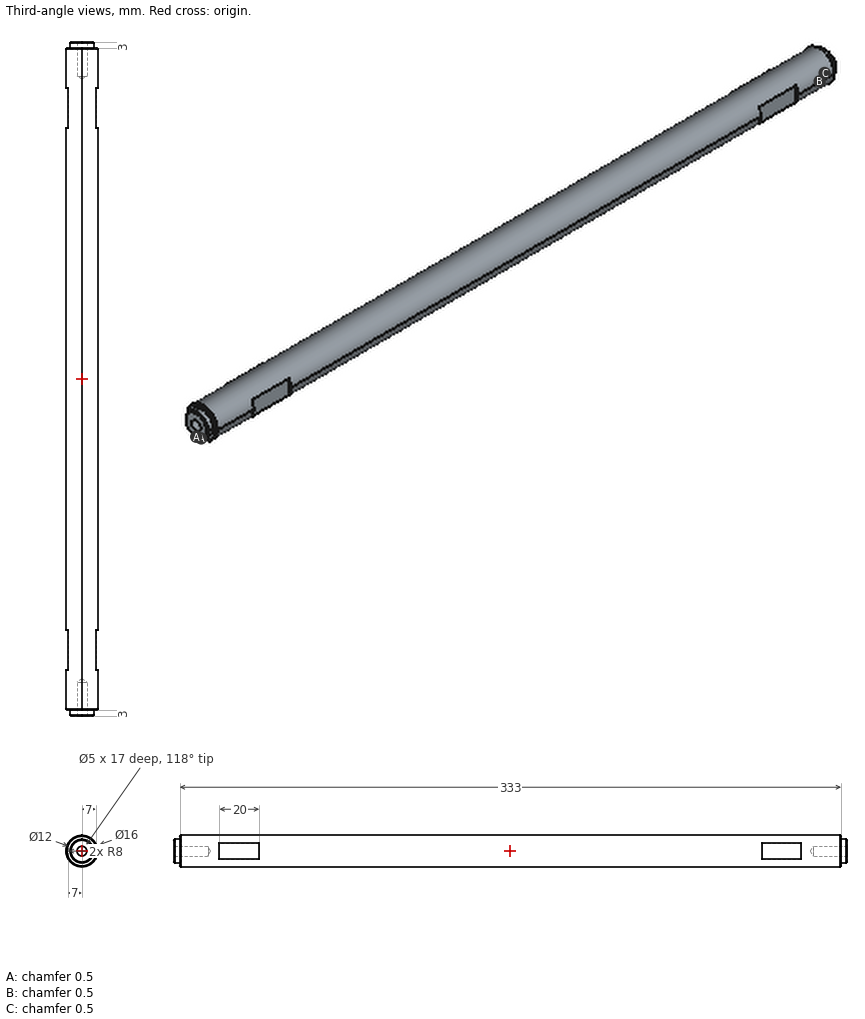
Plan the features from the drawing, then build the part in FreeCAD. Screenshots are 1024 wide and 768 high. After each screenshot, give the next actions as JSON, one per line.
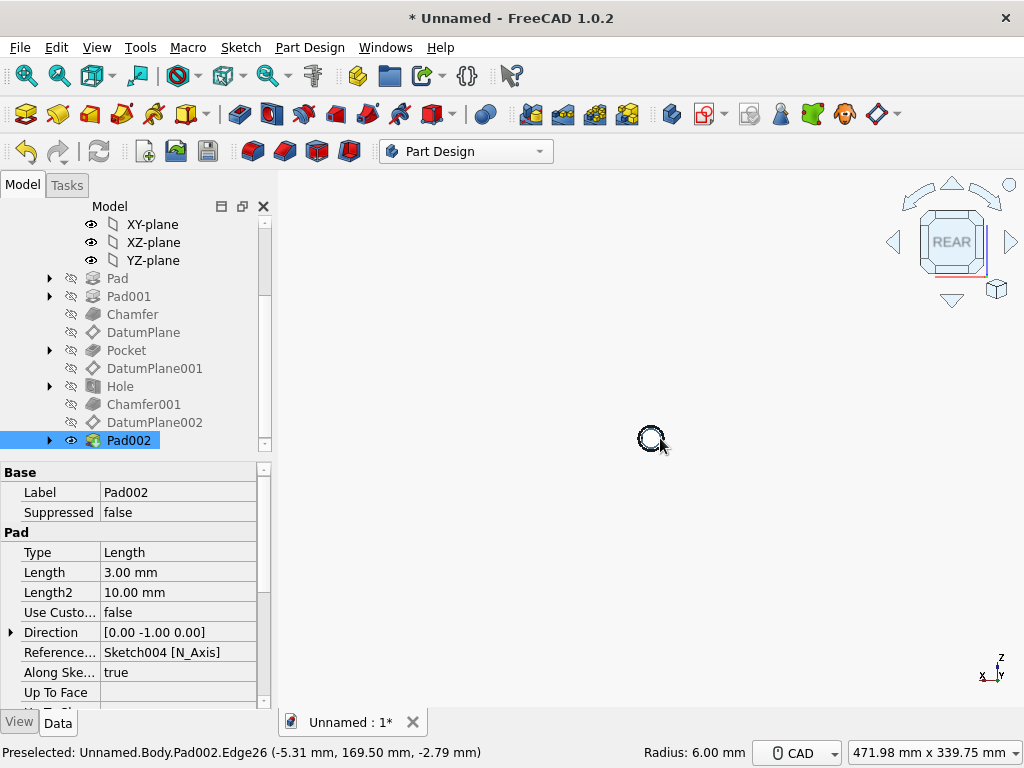
{"action": "left_click", "coordinate": [286, 152]}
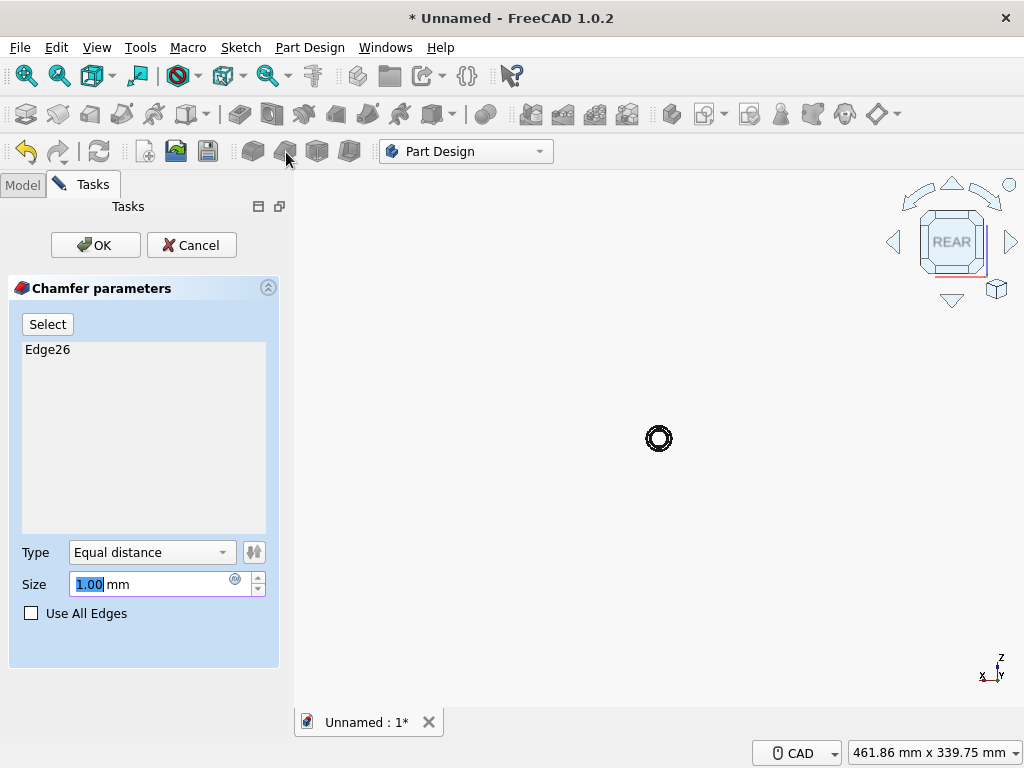
{"action": "type", "text": "0.5"}
{"action": "key", "text": "Tab"}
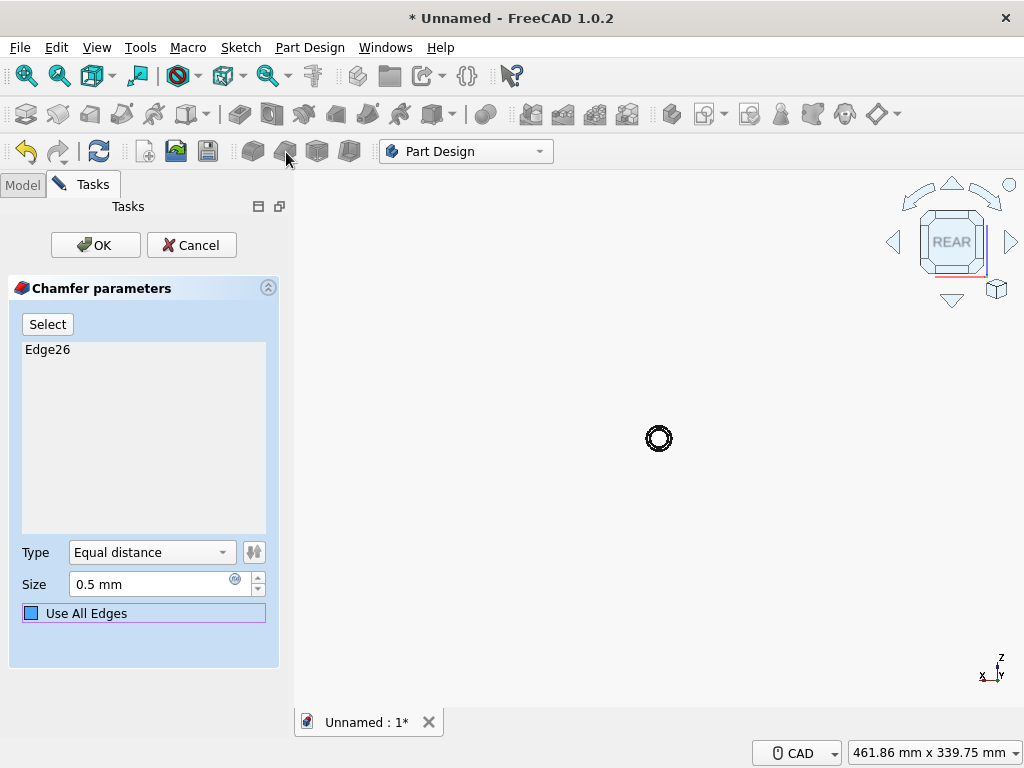
{"action": "left_click", "coordinate": [96, 245]}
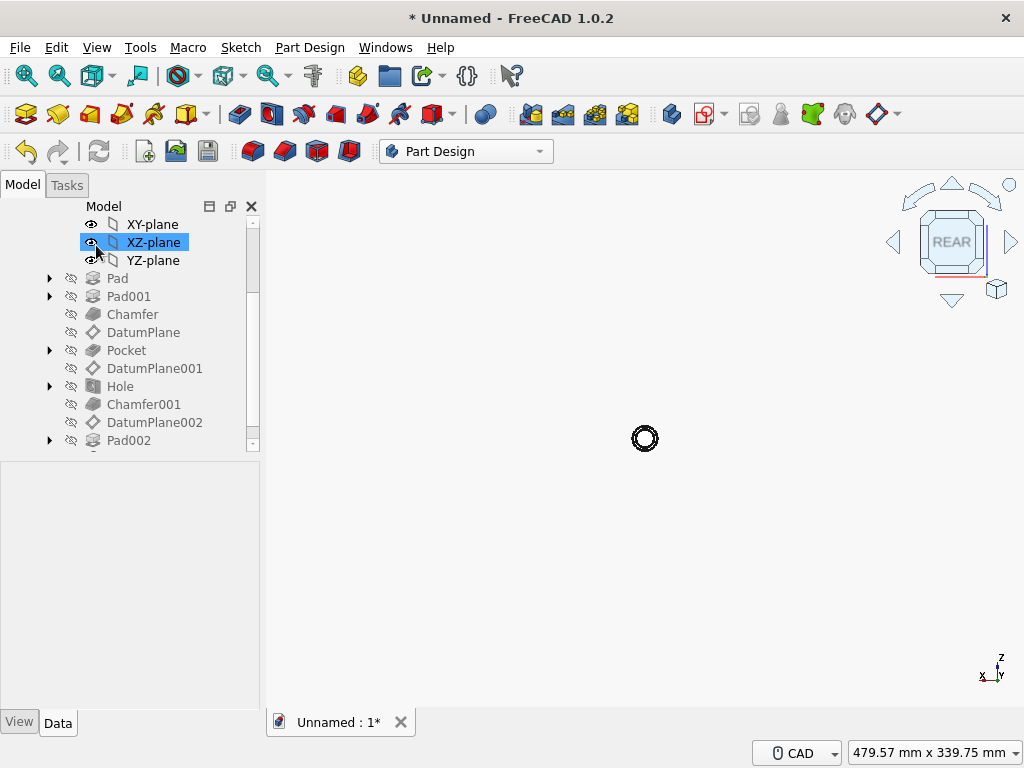
{"action": "key", "text": "v f"}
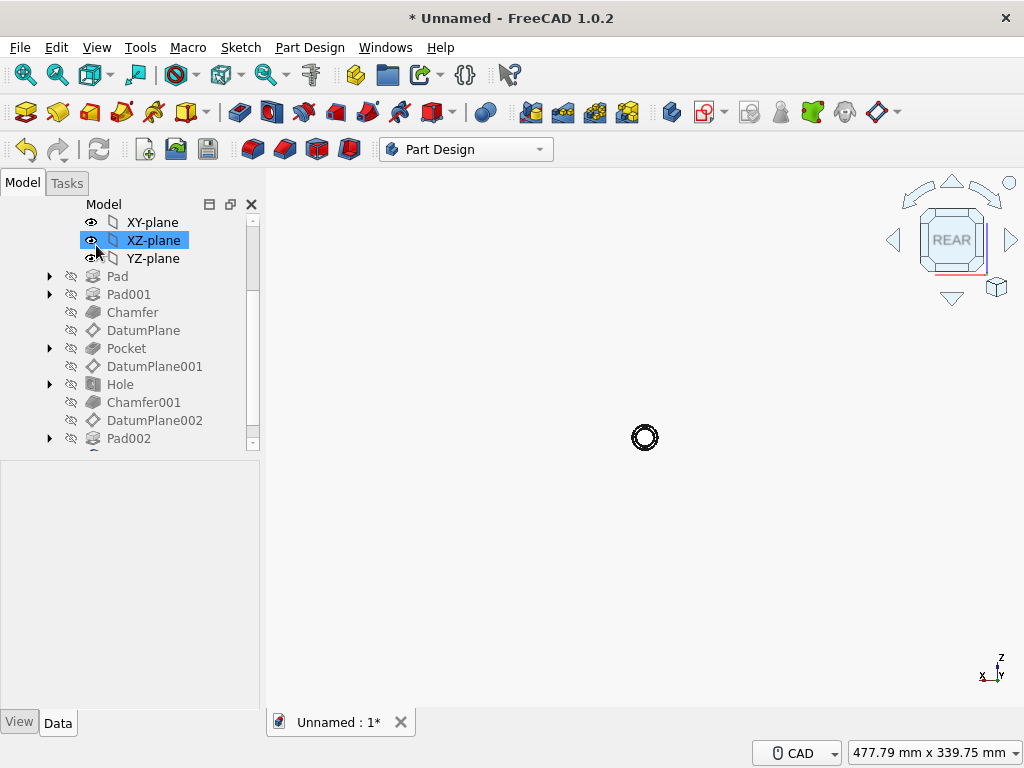
{"action": "key", "text": "5"}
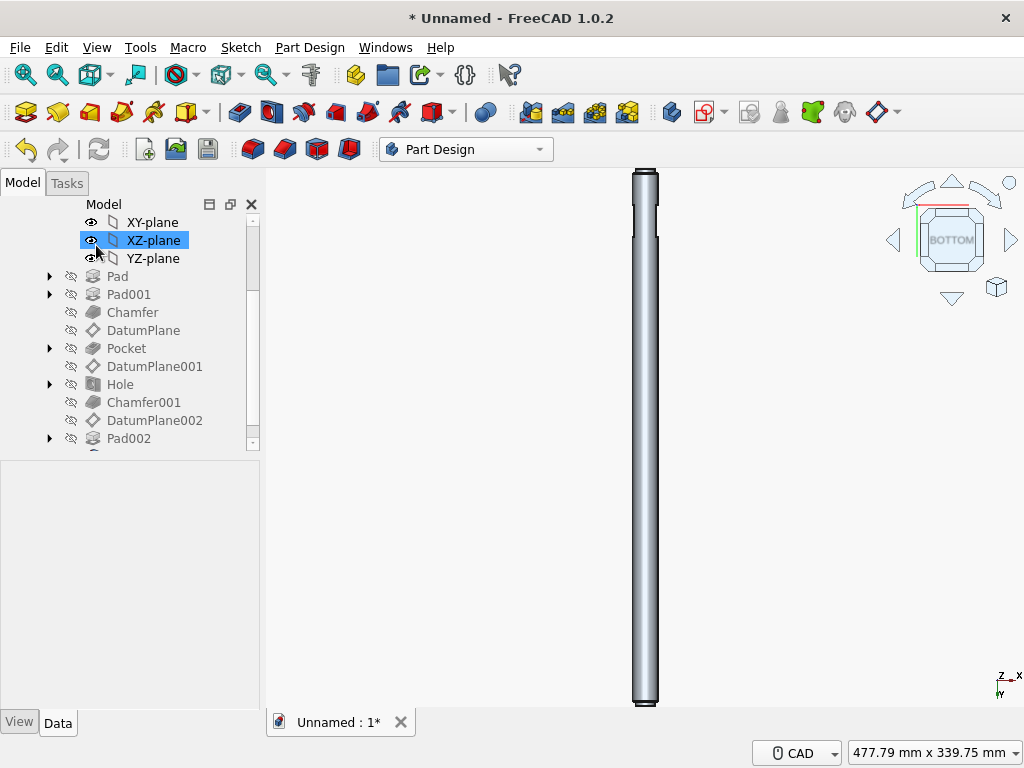
{"action": "key", "text": "4"}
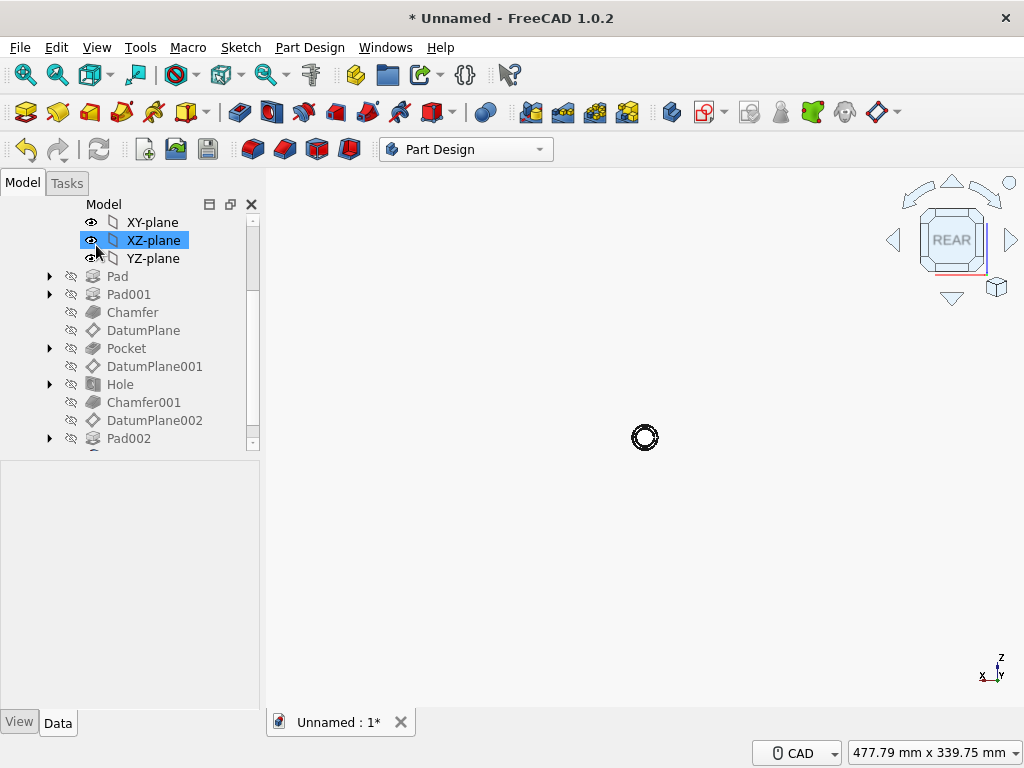
{"action": "key", "text": "v f"}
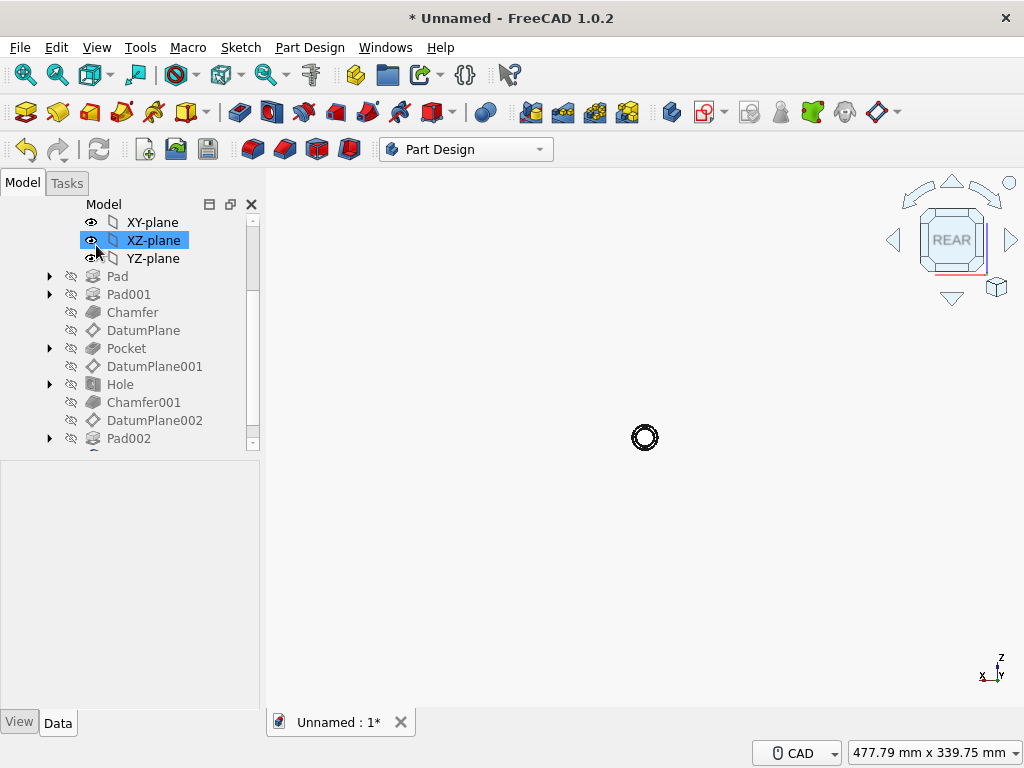
{"action": "key", "text": "3"}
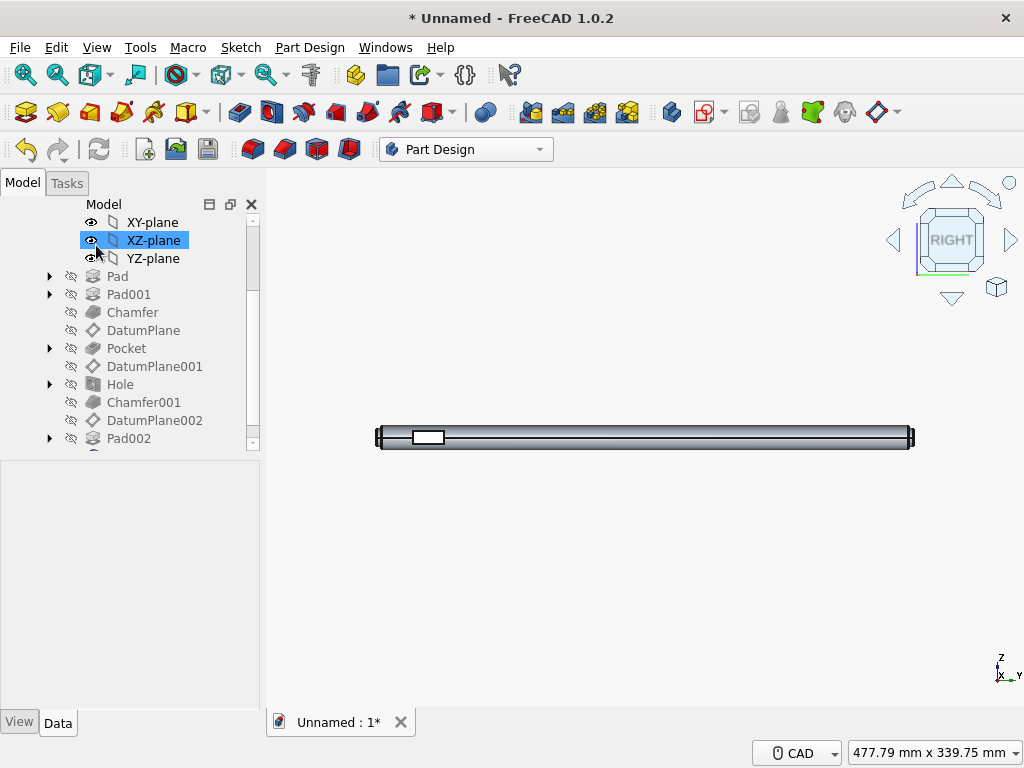
{"action": "scroll", "coordinate": [160, 326], "scroll_direction": "down", "scroll_amount": 3}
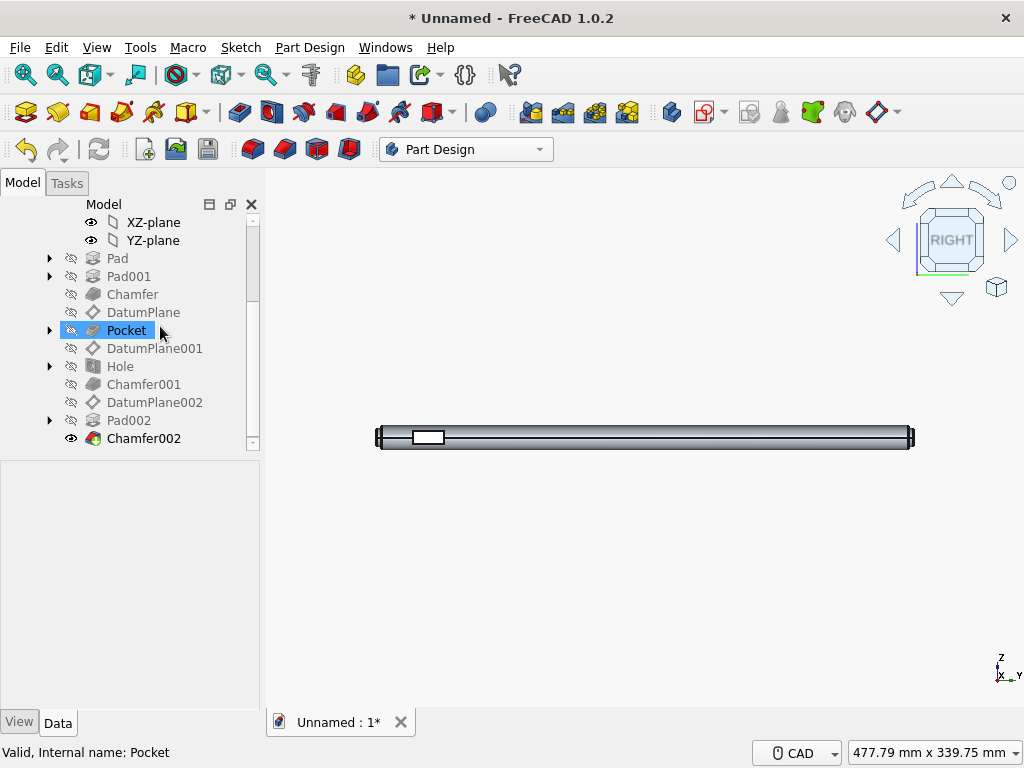
{"action": "scroll", "coordinate": [160, 326], "scroll_direction": "up", "scroll_amount": 15}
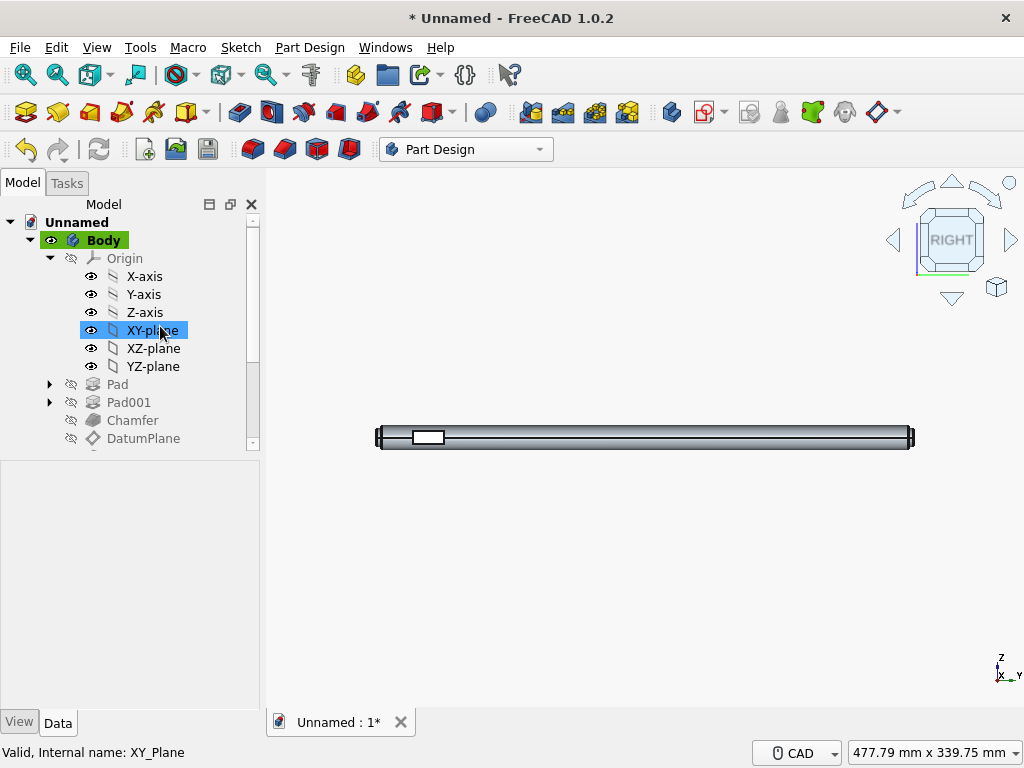
{"action": "left_click", "coordinate": [136, 348]}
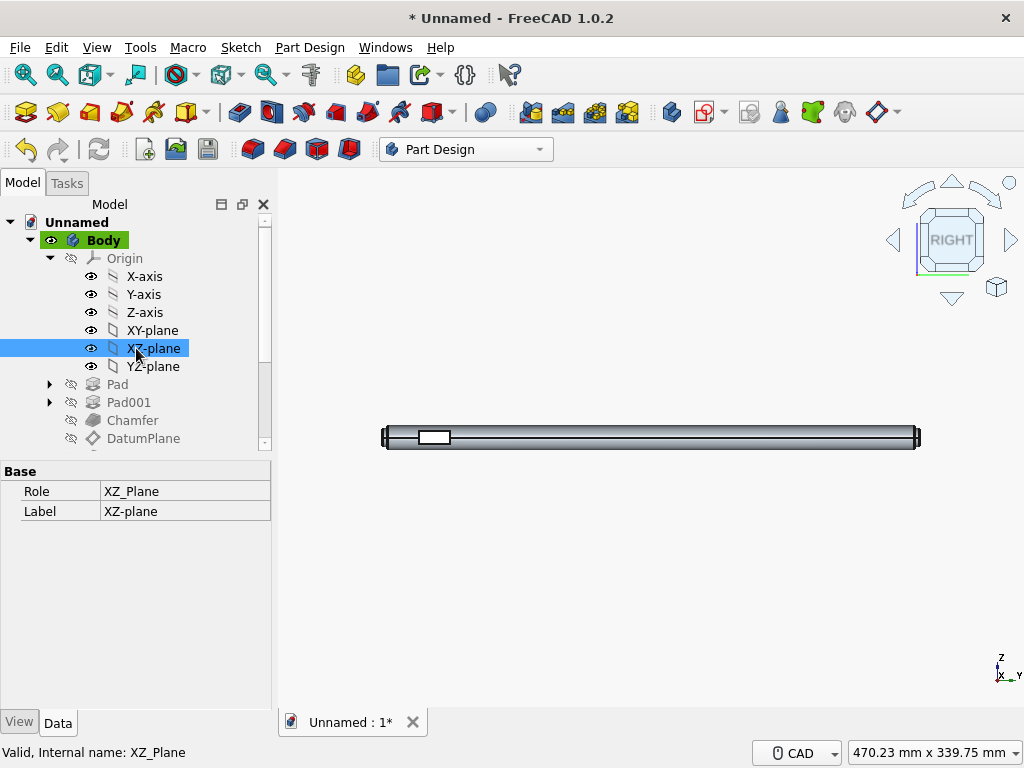
{"action": "left_click", "coordinate": [878, 112]}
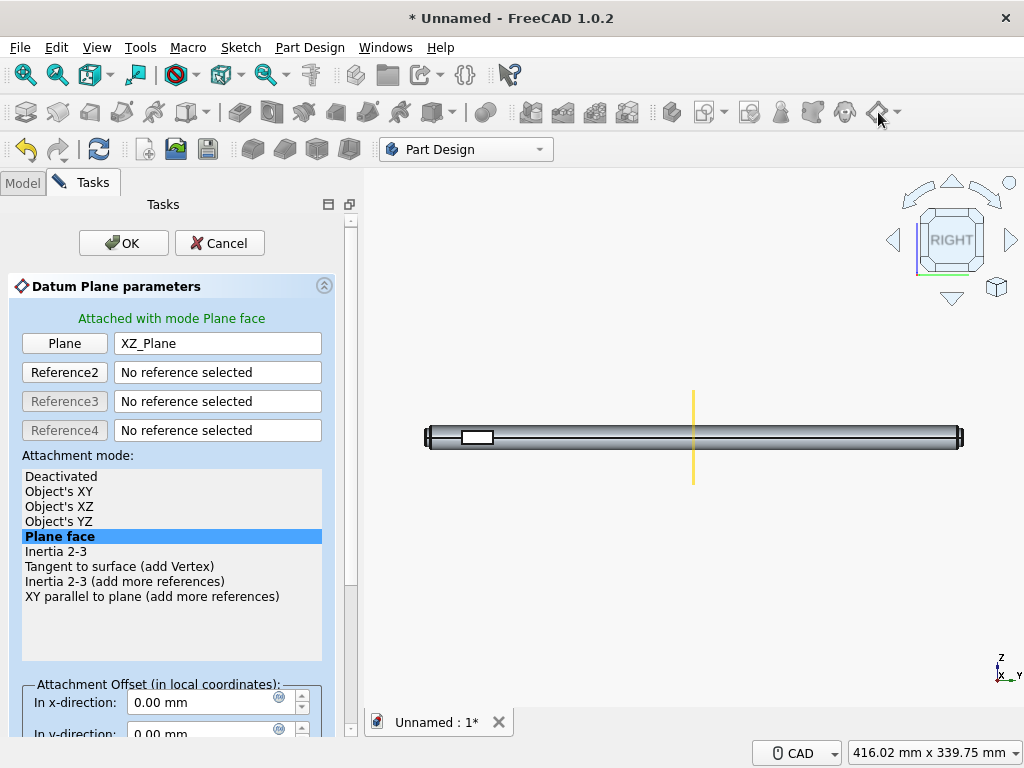
{"action": "scroll", "coordinate": [351, 475], "scroll_direction": "down", "scroll_amount": 2}